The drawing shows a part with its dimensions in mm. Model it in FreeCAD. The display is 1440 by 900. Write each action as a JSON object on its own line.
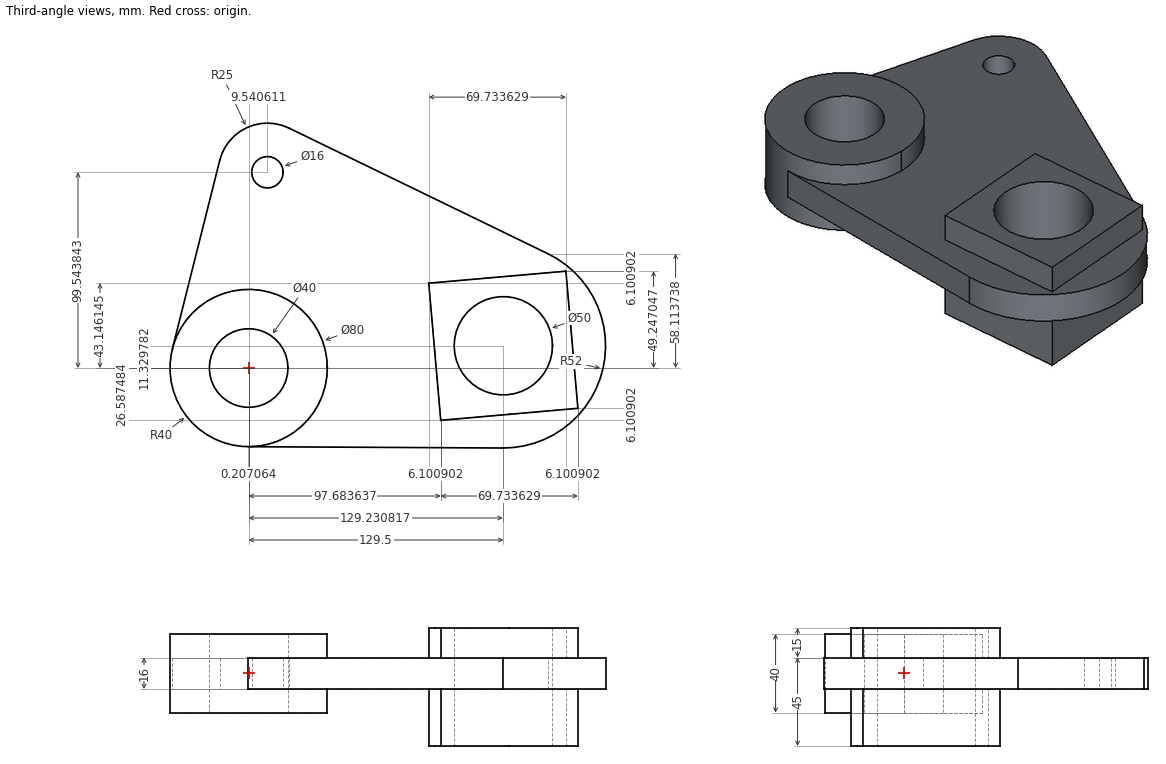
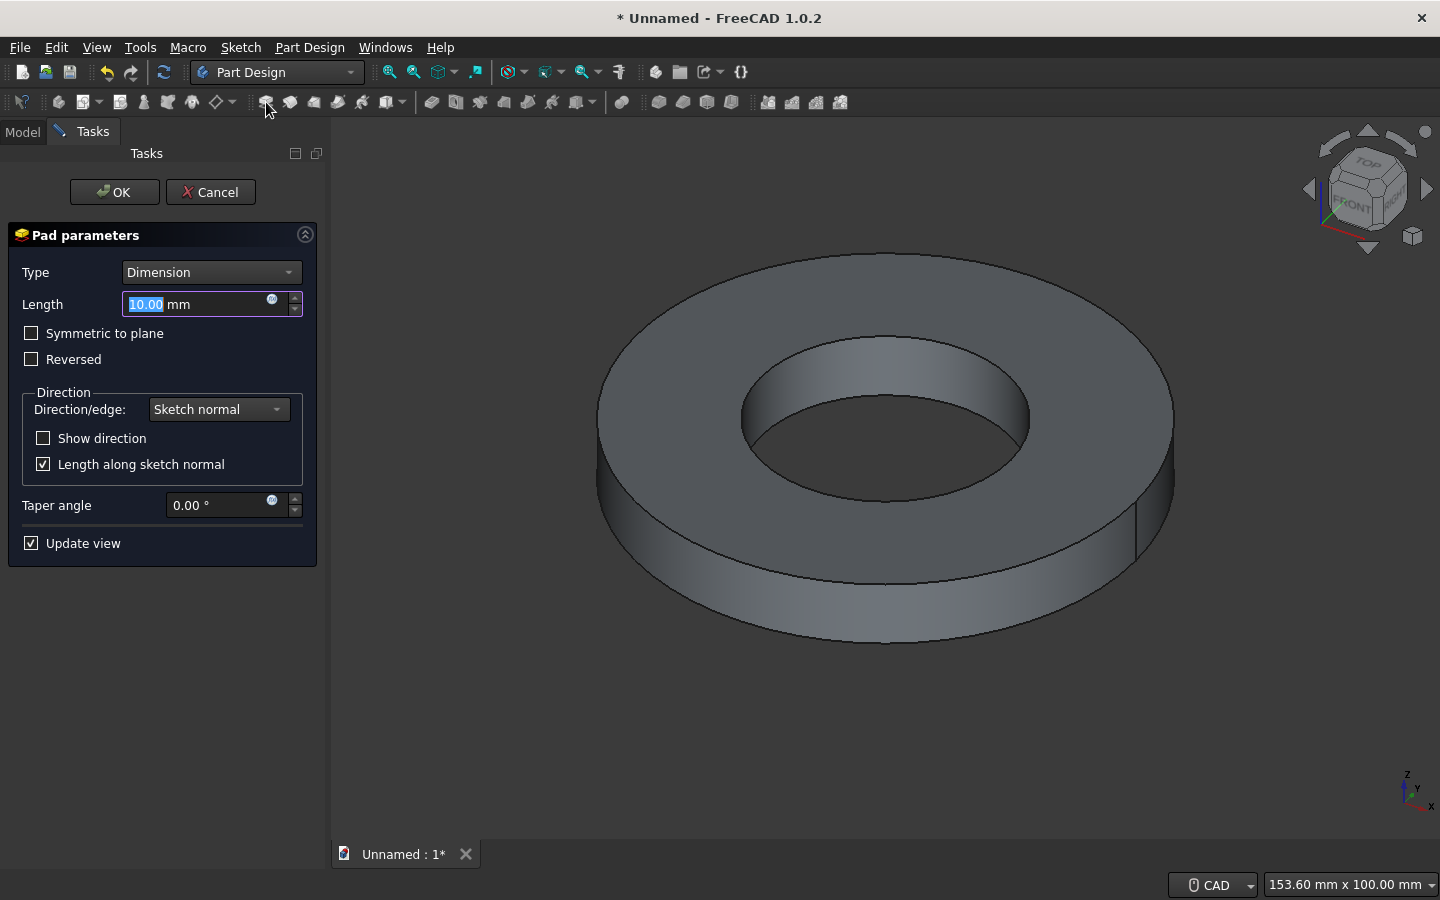
{"action": "type", "text": "40"}
{"action": "key", "text": "Tab"}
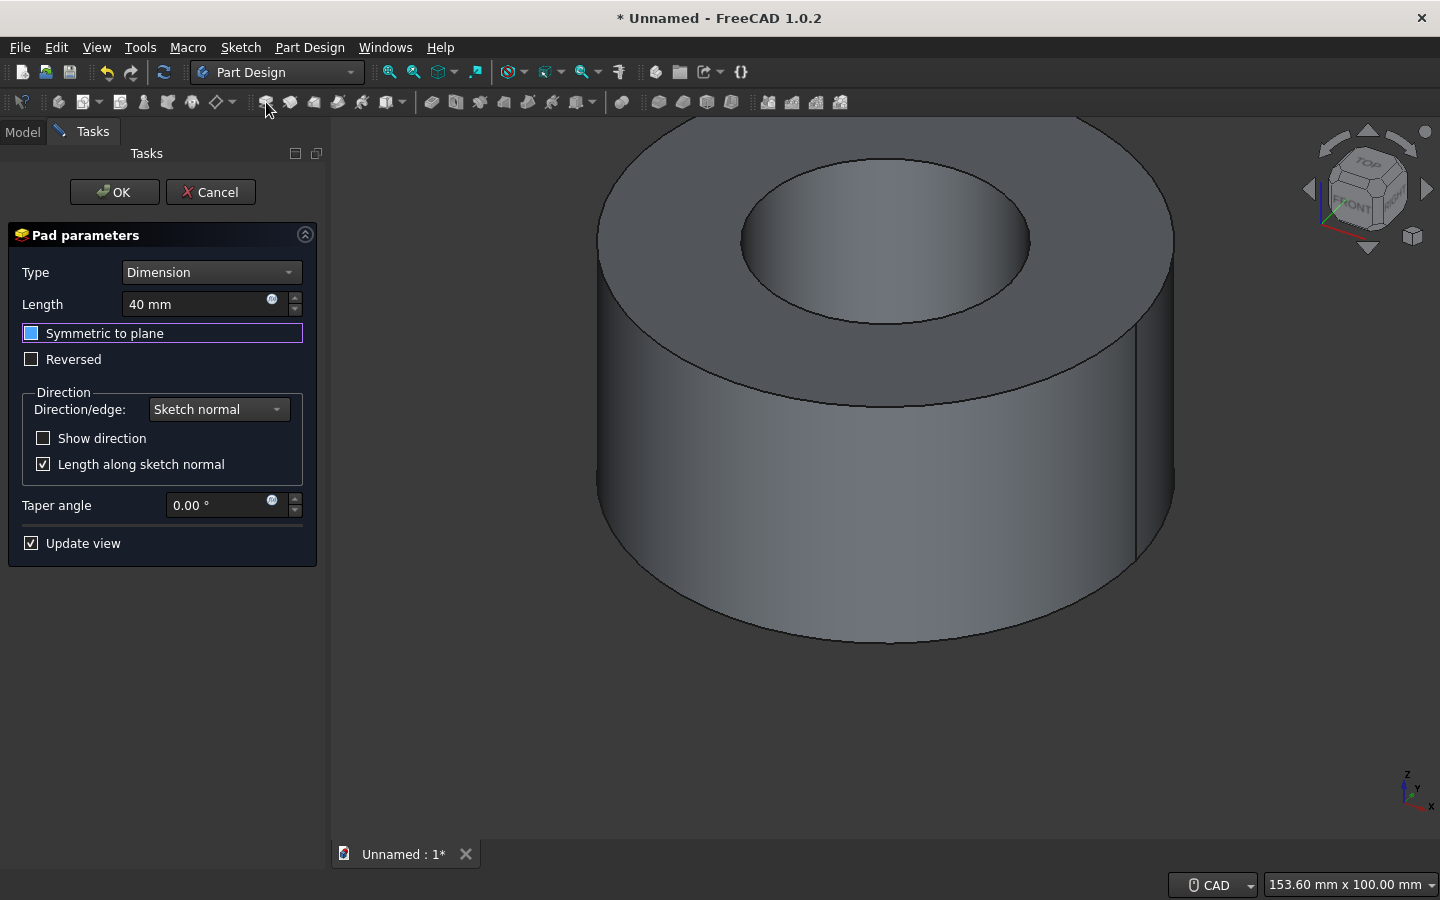
{"action": "left_click", "coordinate": [30, 333]}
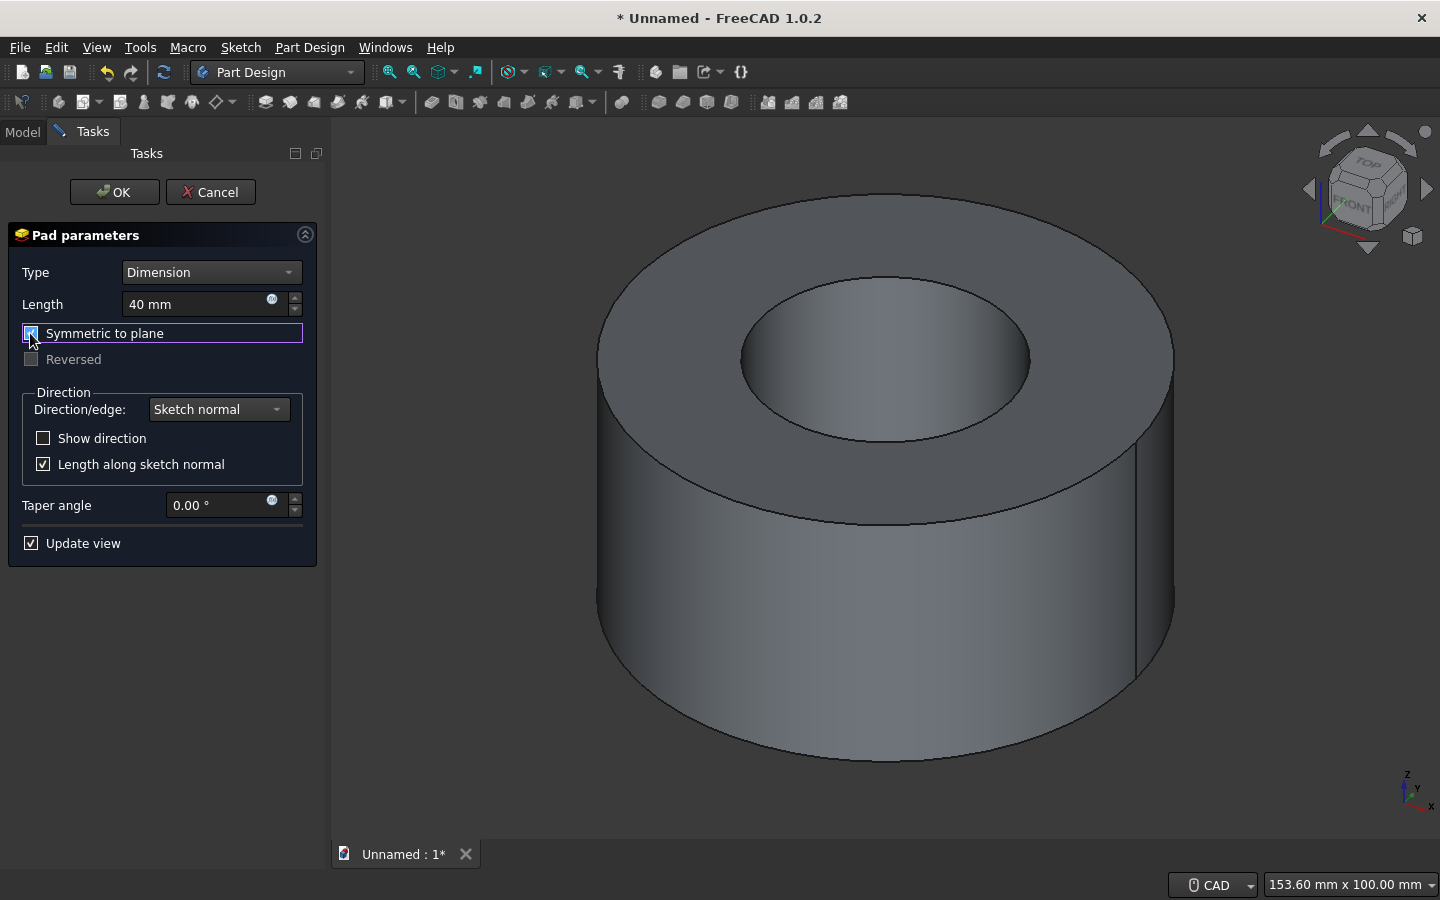
{"action": "left_click", "coordinate": [115, 192]}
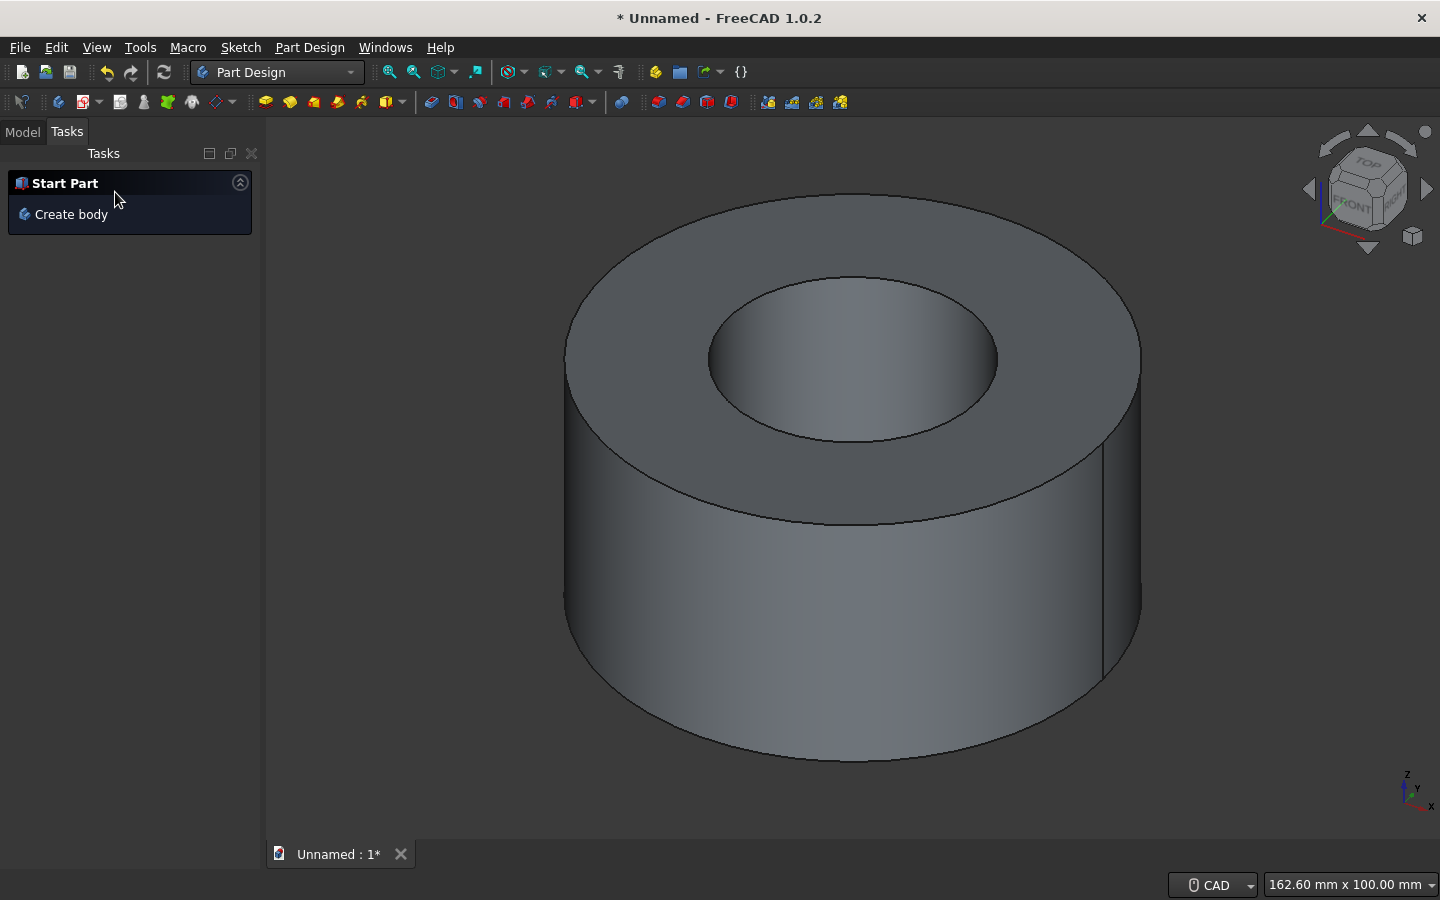
{"action": "left_click", "coordinate": [84, 102]}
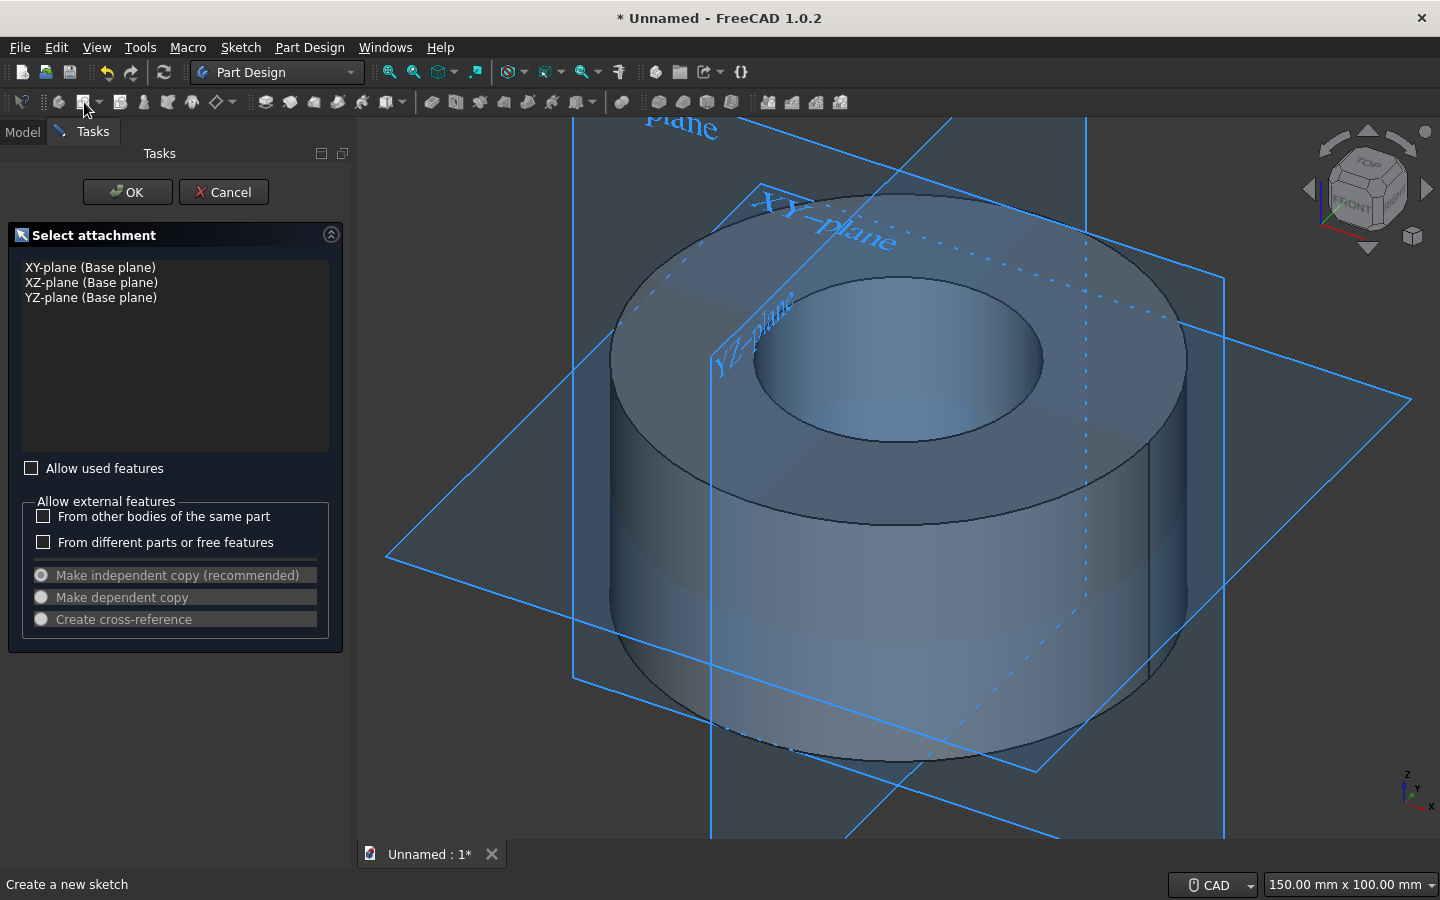
{"action": "left_click", "coordinate": [82, 268]}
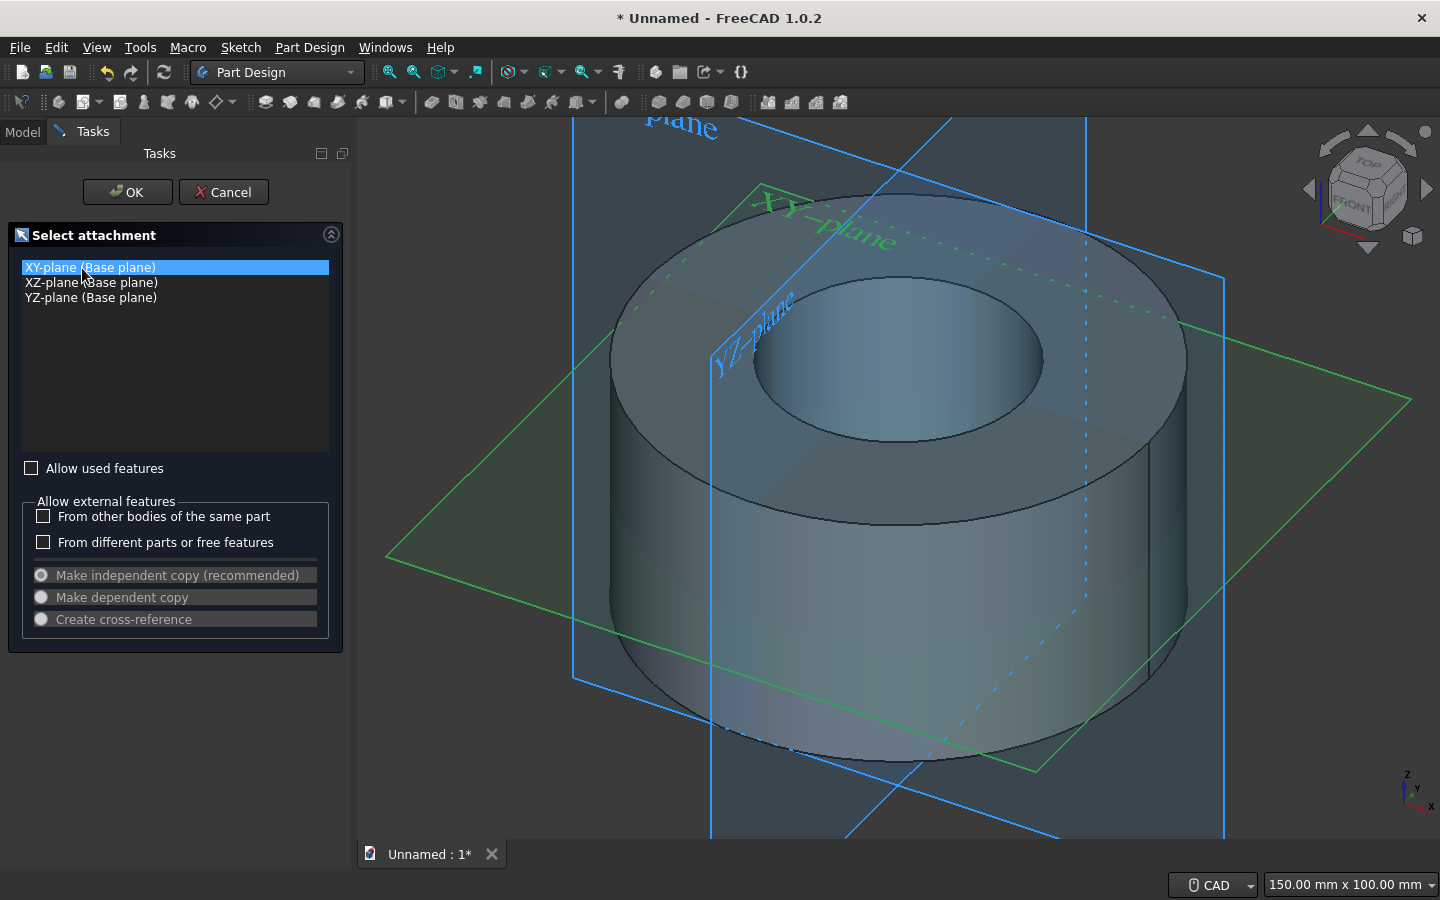
{"action": "left_click", "coordinate": [128, 192]}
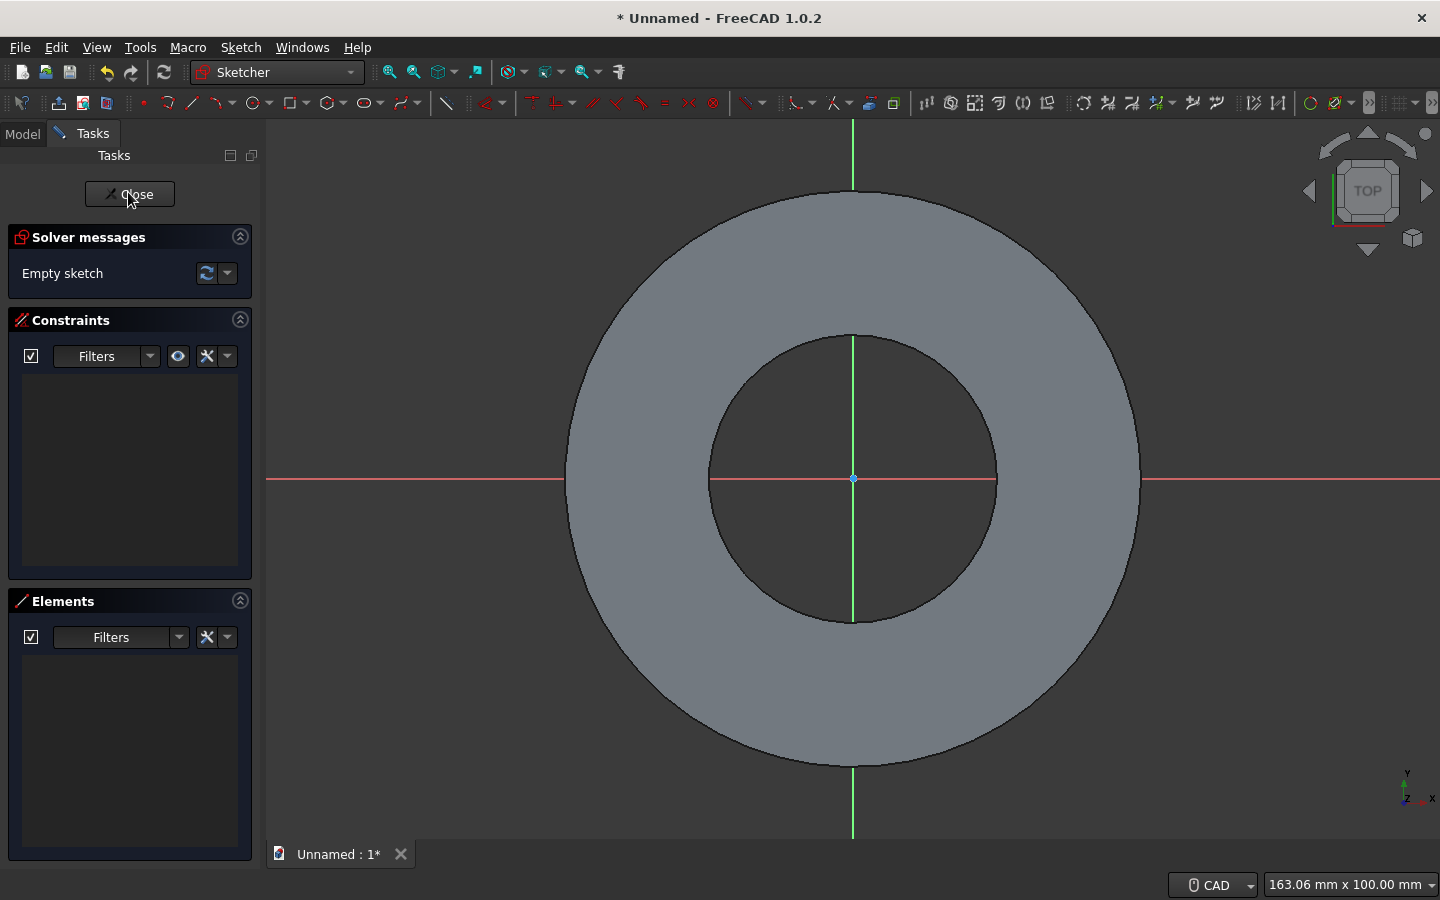
{"action": "left_click", "coordinate": [108, 104]}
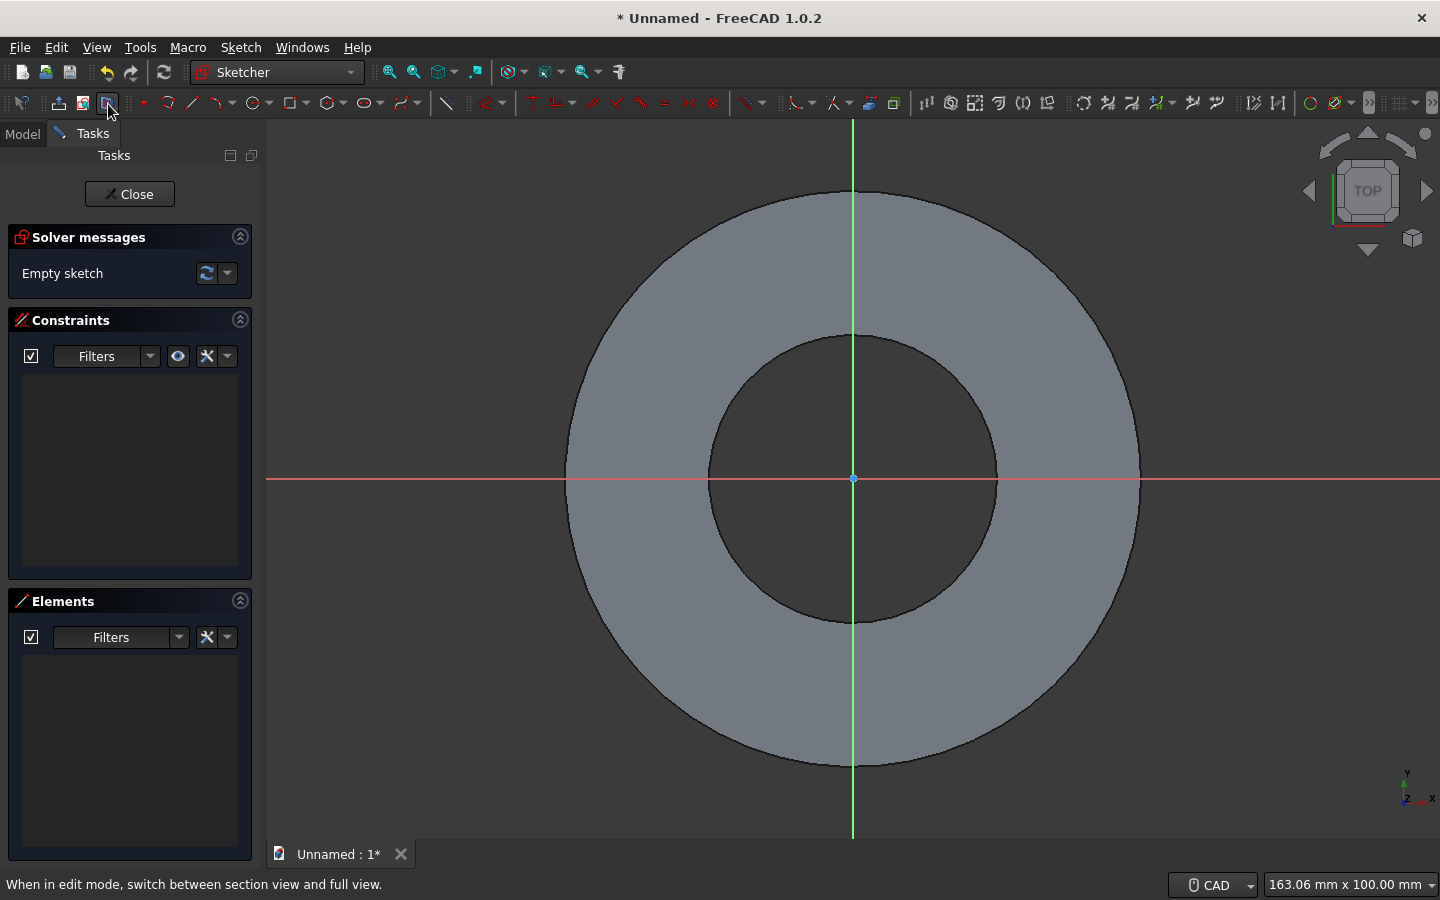
{"action": "scroll", "coordinate": [448, 650], "scroll_direction": "down", "scroll_amount": 5}